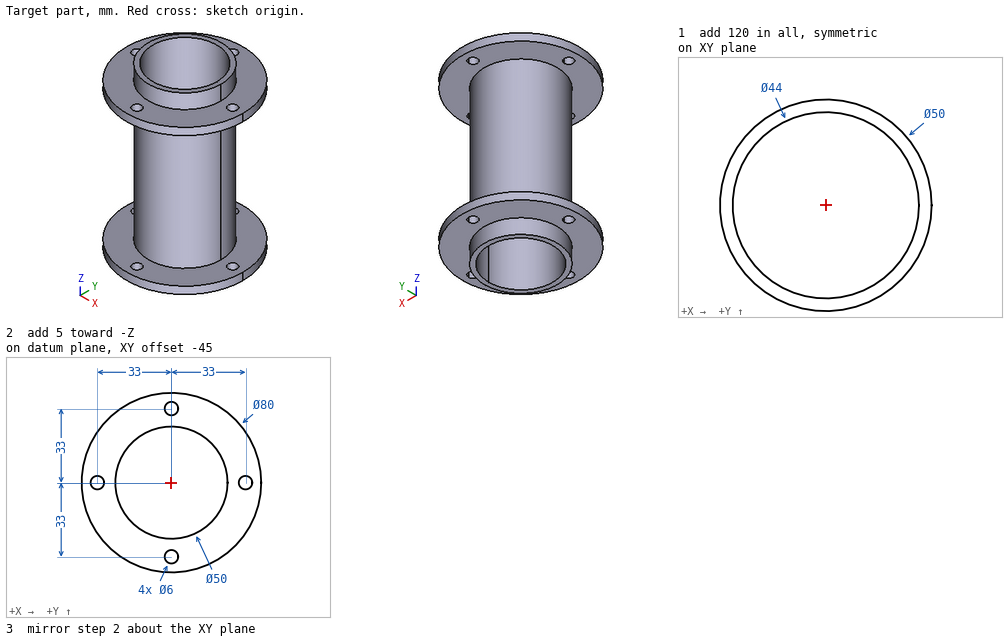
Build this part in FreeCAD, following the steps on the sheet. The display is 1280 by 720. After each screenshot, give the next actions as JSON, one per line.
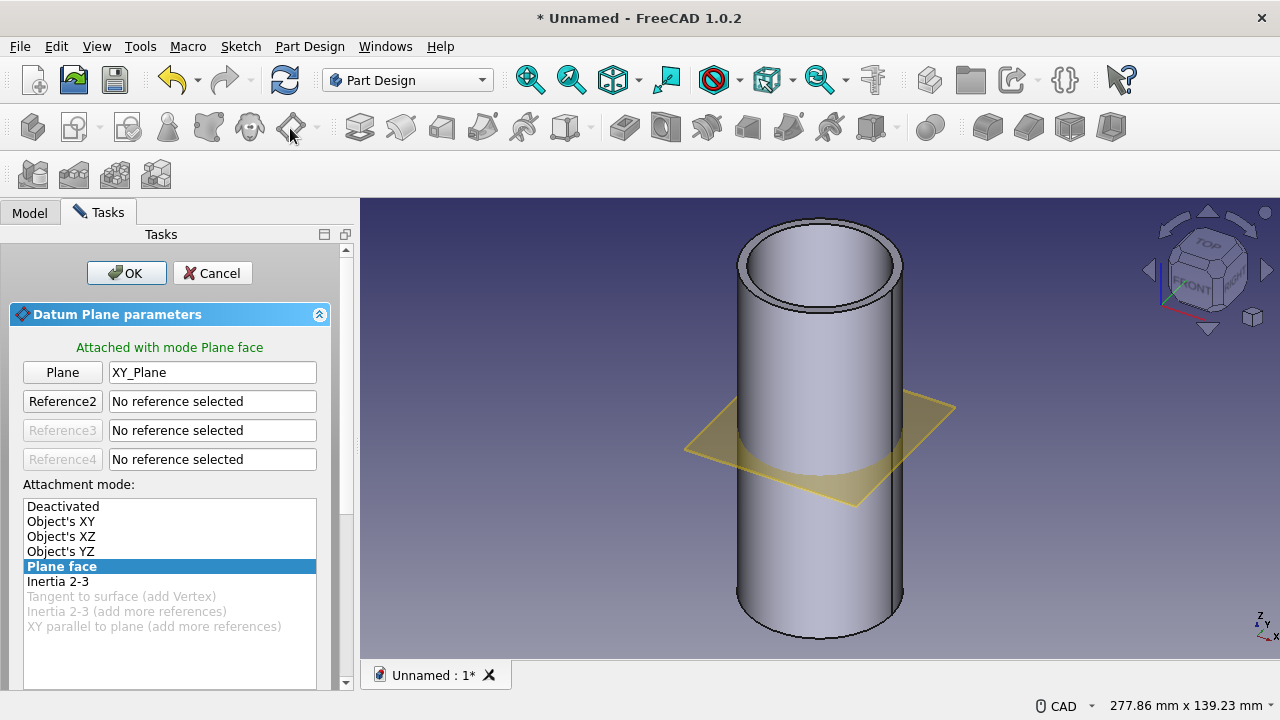
{"action": "scroll", "coordinate": [346, 467], "scroll_direction": "down", "scroll_amount": 4}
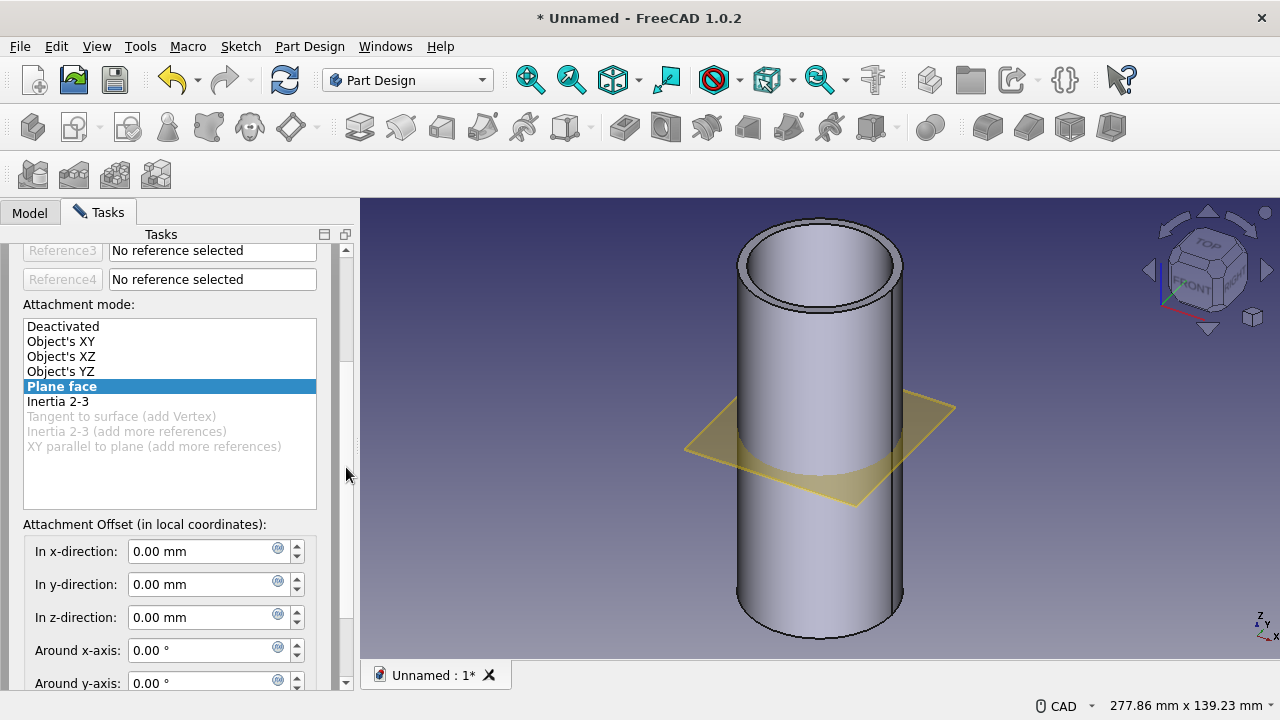
{"action": "triple_click", "coordinate": [210, 558]}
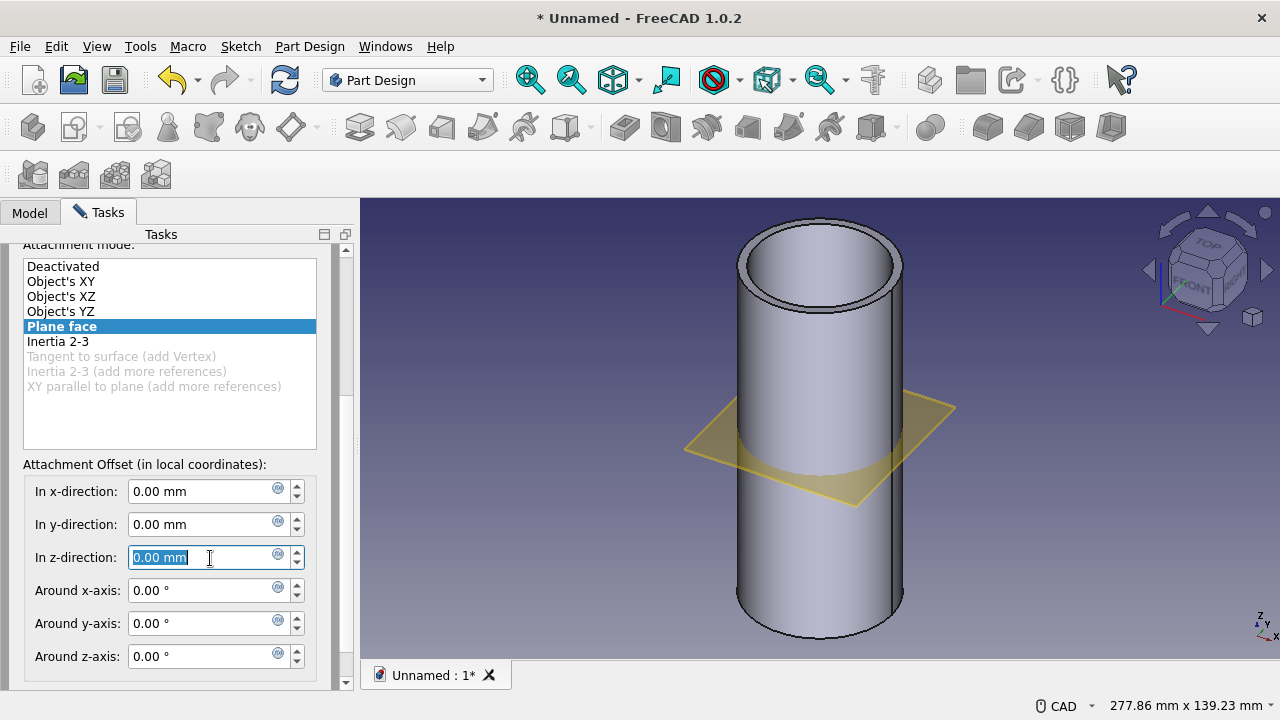
{"action": "type", "text": "-45"}
{"action": "key", "text": "Tab"}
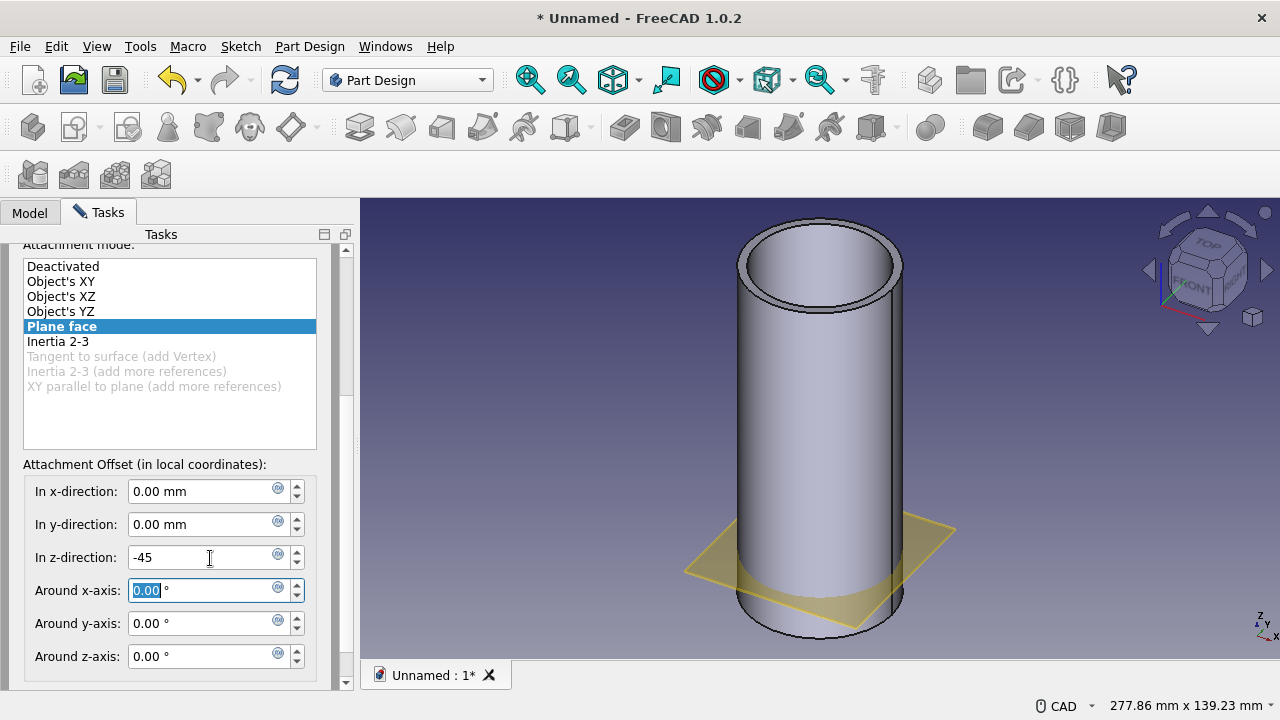
{"action": "scroll", "coordinate": [346, 467], "scroll_direction": "up", "scroll_amount": 5}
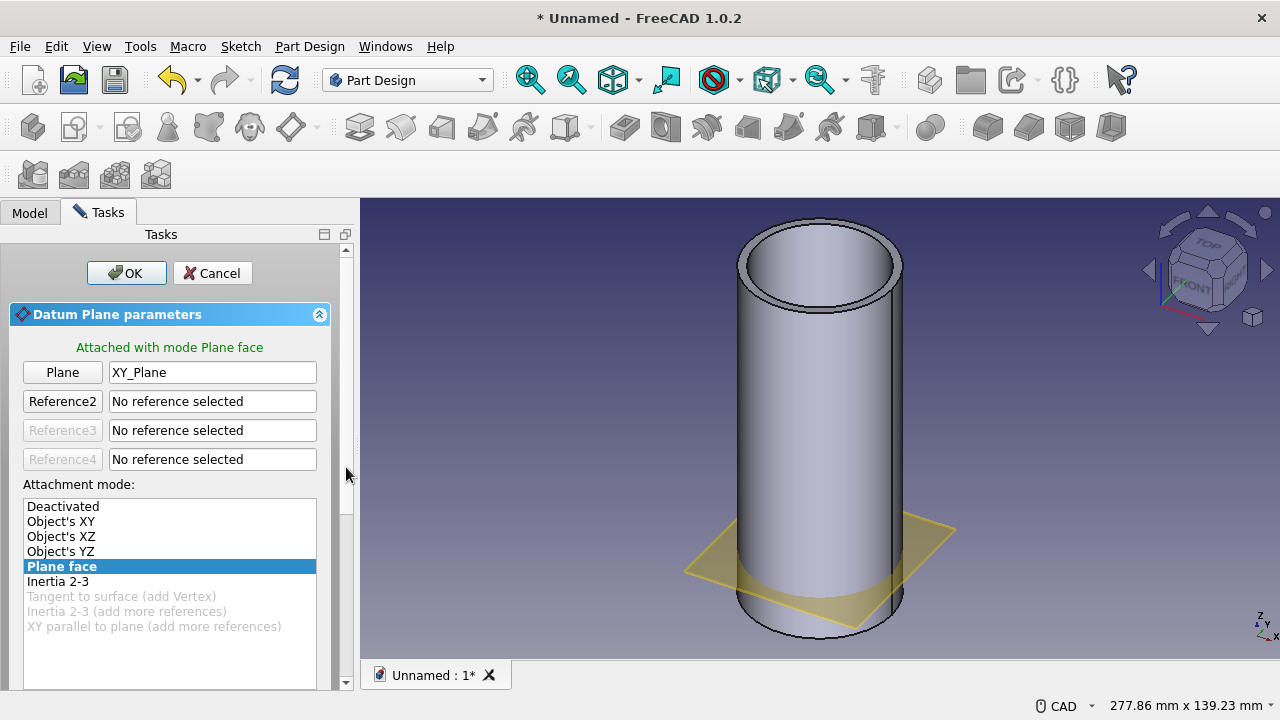
{"action": "left_click", "coordinate": [127, 273]}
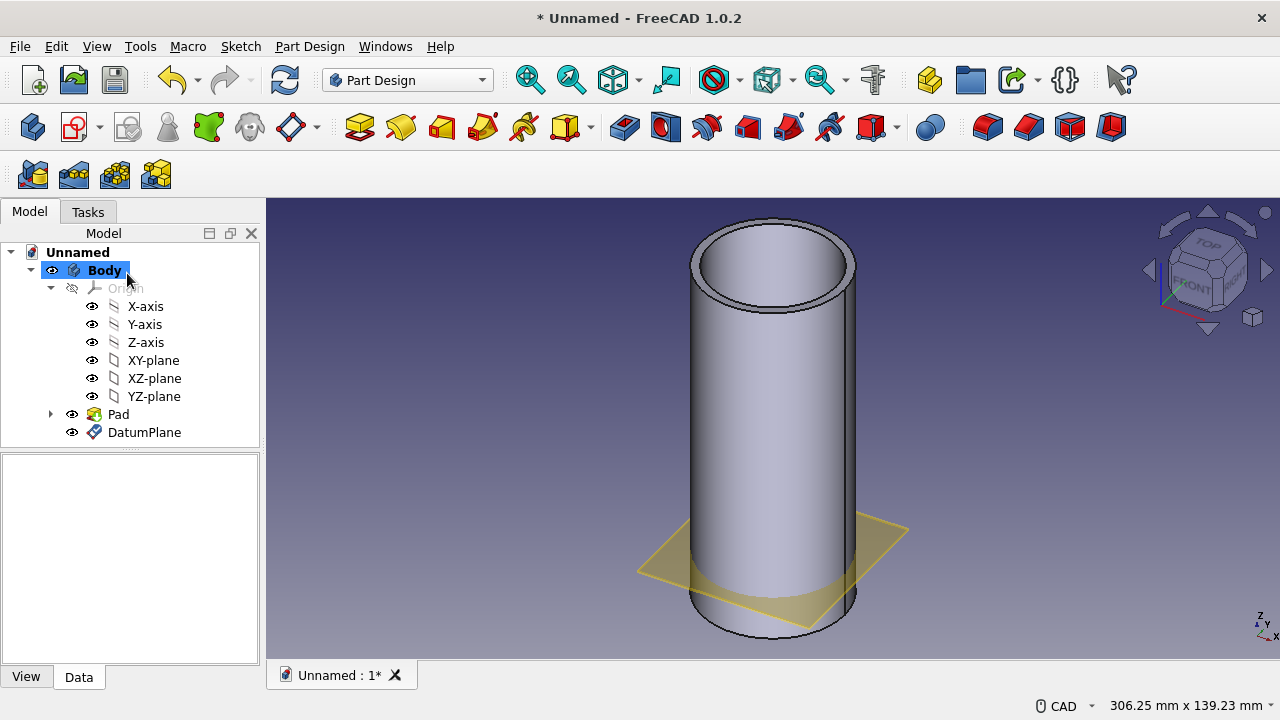
{"action": "left_click", "coordinate": [117, 432]}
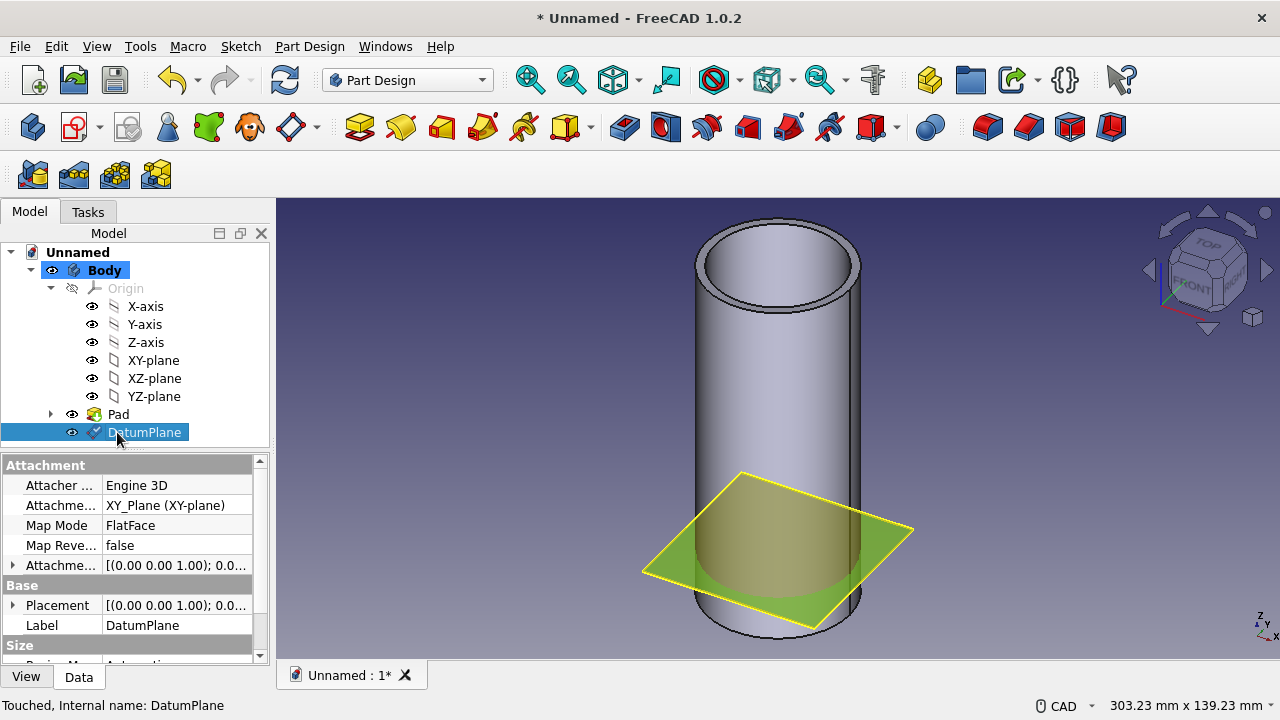
{"action": "left_click", "coordinate": [74, 128]}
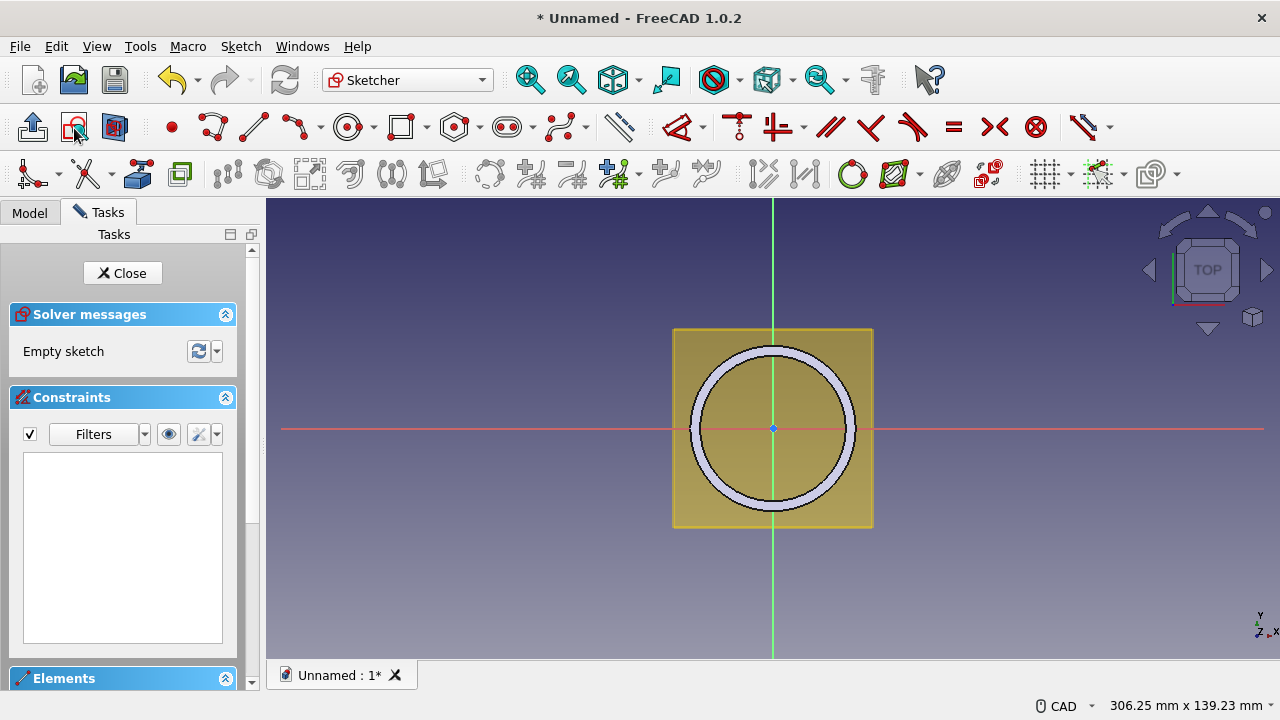
{"action": "left_click", "coordinate": [115, 128]}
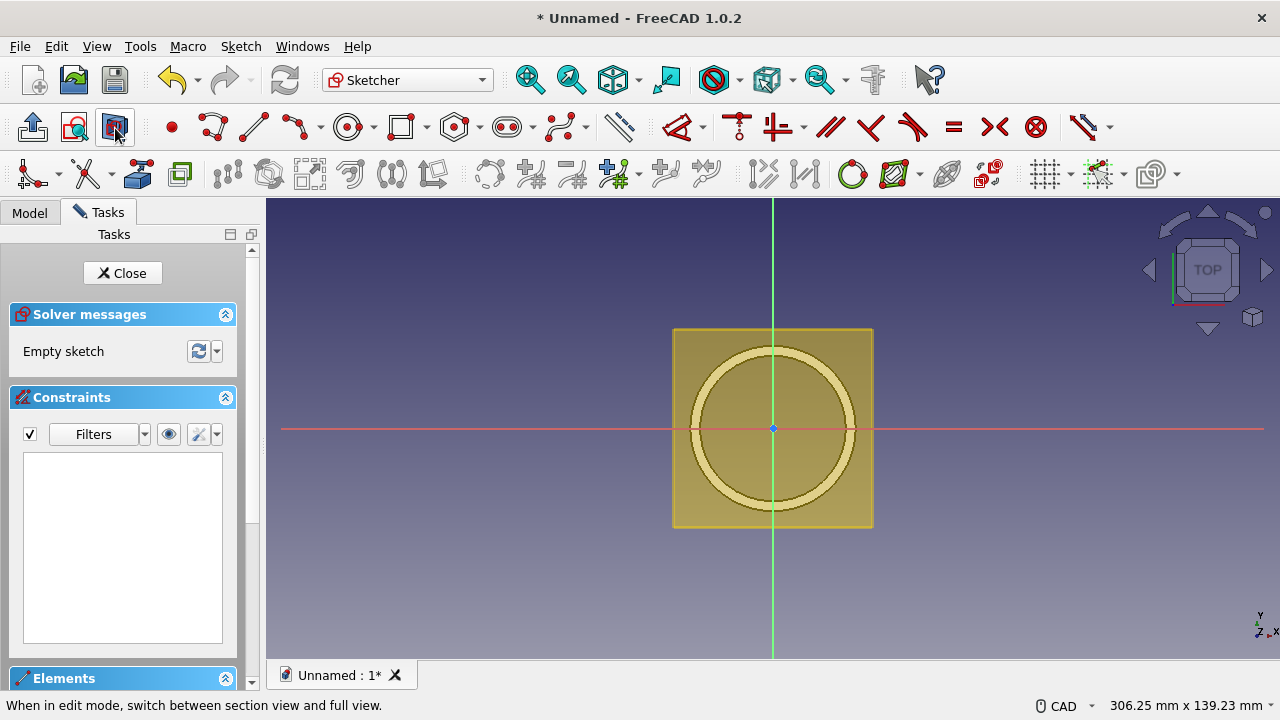
{"action": "left_click", "coordinate": [348, 128]}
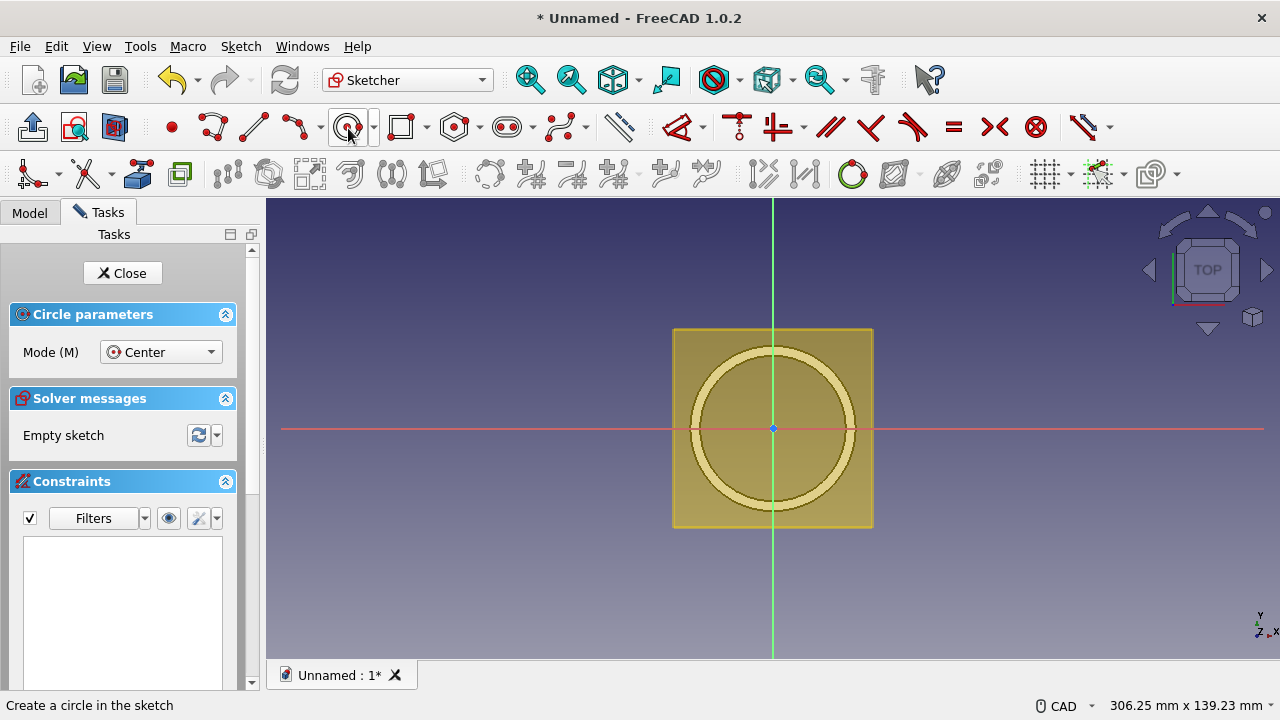
{"action": "left_click", "coordinate": [773, 428]}
{"action": "left_click", "coordinate": [867, 335]}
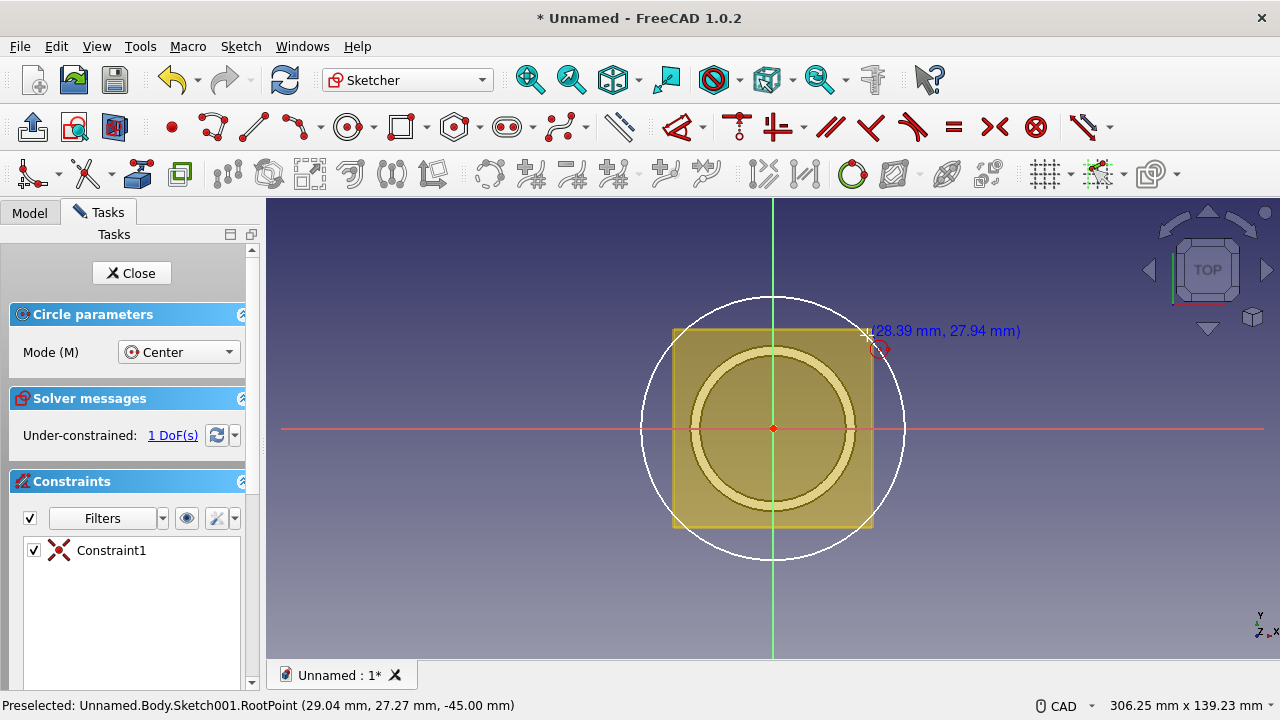
{"action": "scroll", "coordinate": [773, 538], "scroll_direction": "up", "scroll_amount": 5}